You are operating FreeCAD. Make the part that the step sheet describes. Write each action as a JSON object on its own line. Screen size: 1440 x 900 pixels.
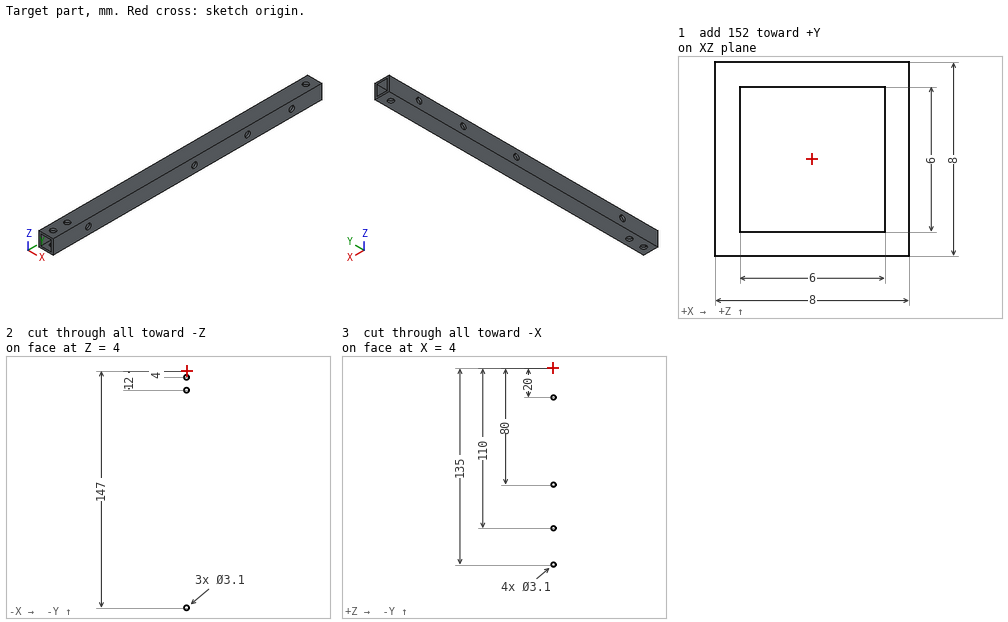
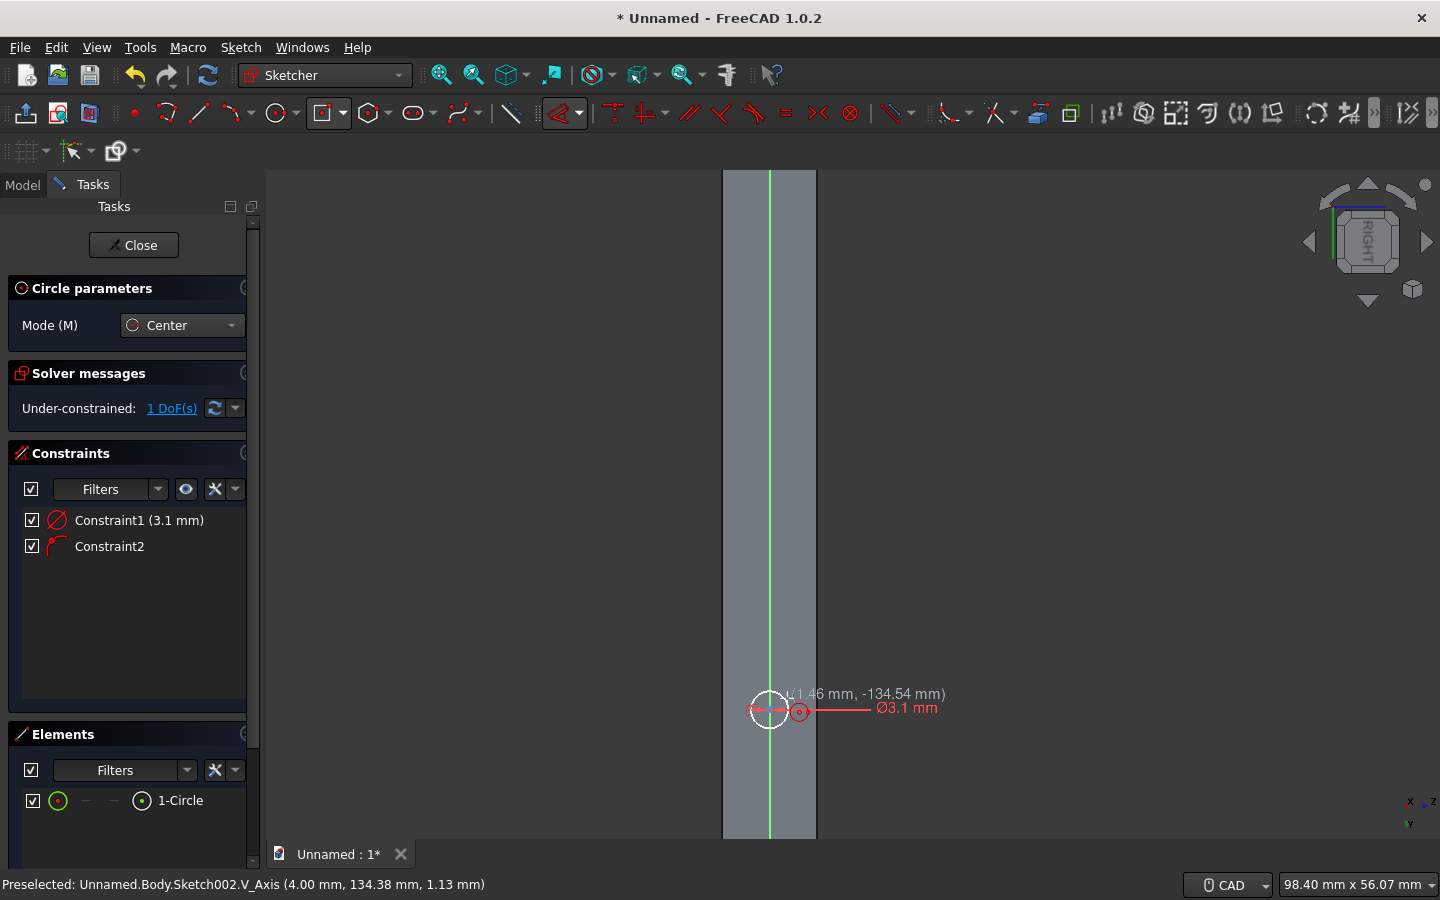
{"action": "scroll", "coordinate": [789, 700], "scroll_direction": "down", "scroll_amount": 7}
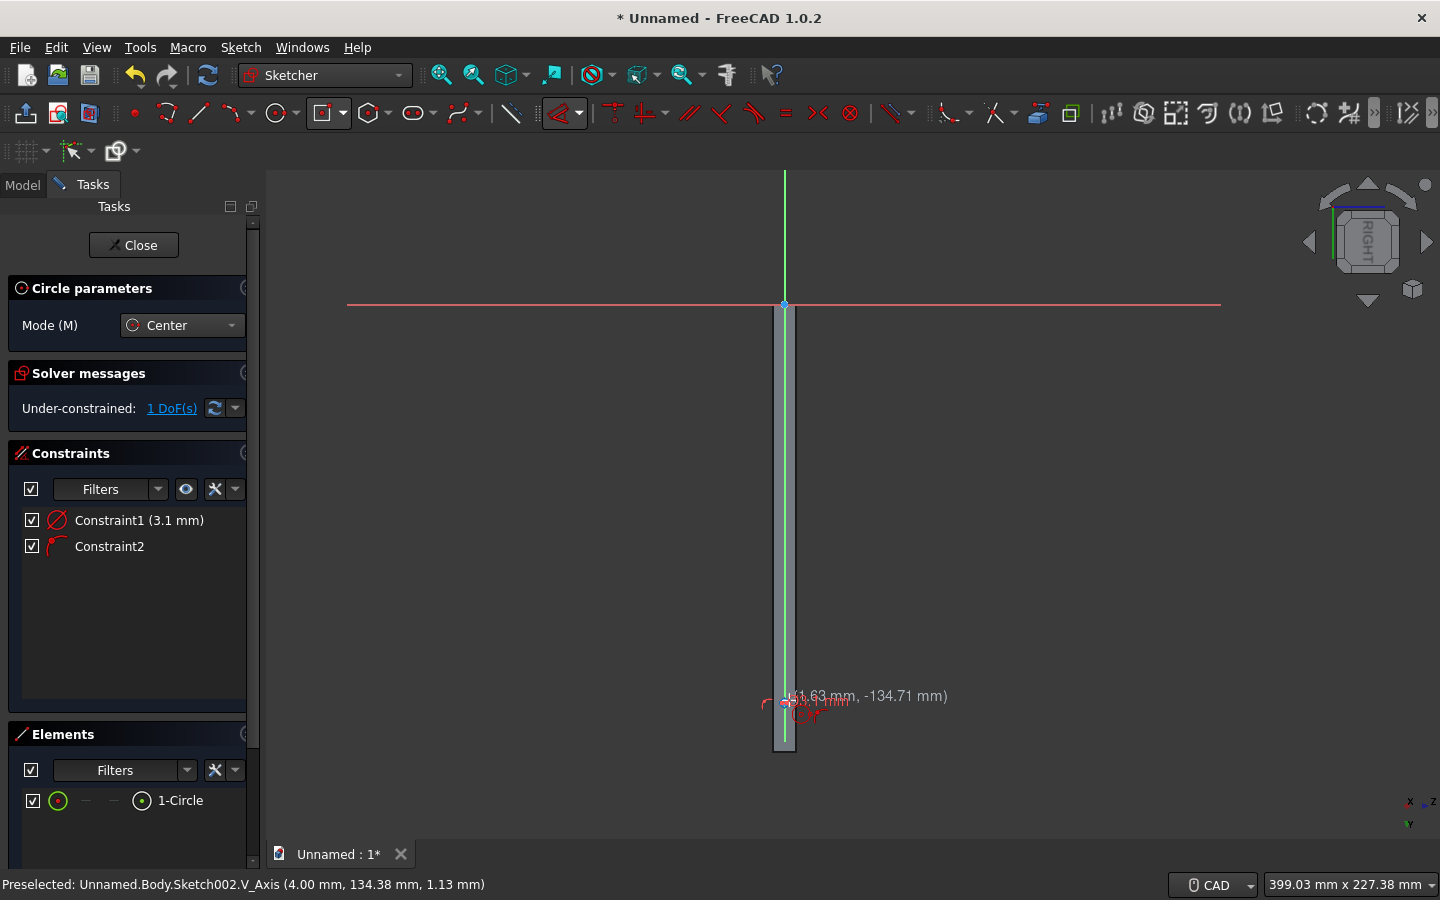
{"action": "scroll", "coordinate": [785, 363], "scroll_direction": "up", "scroll_amount": 9}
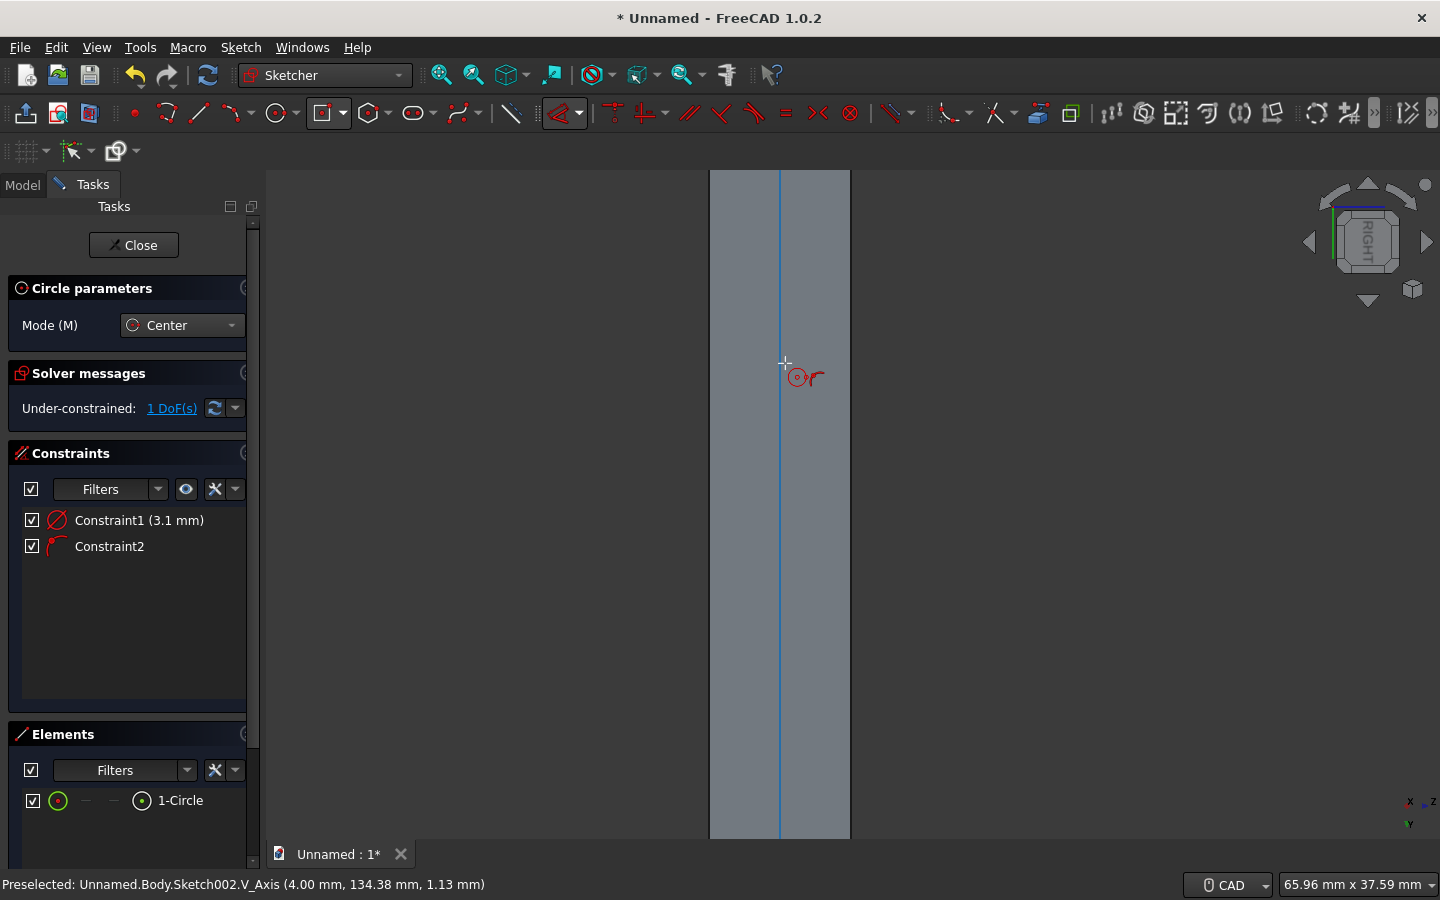
{"action": "scroll", "coordinate": [785, 362], "scroll_direction": "down", "scroll_amount": 9}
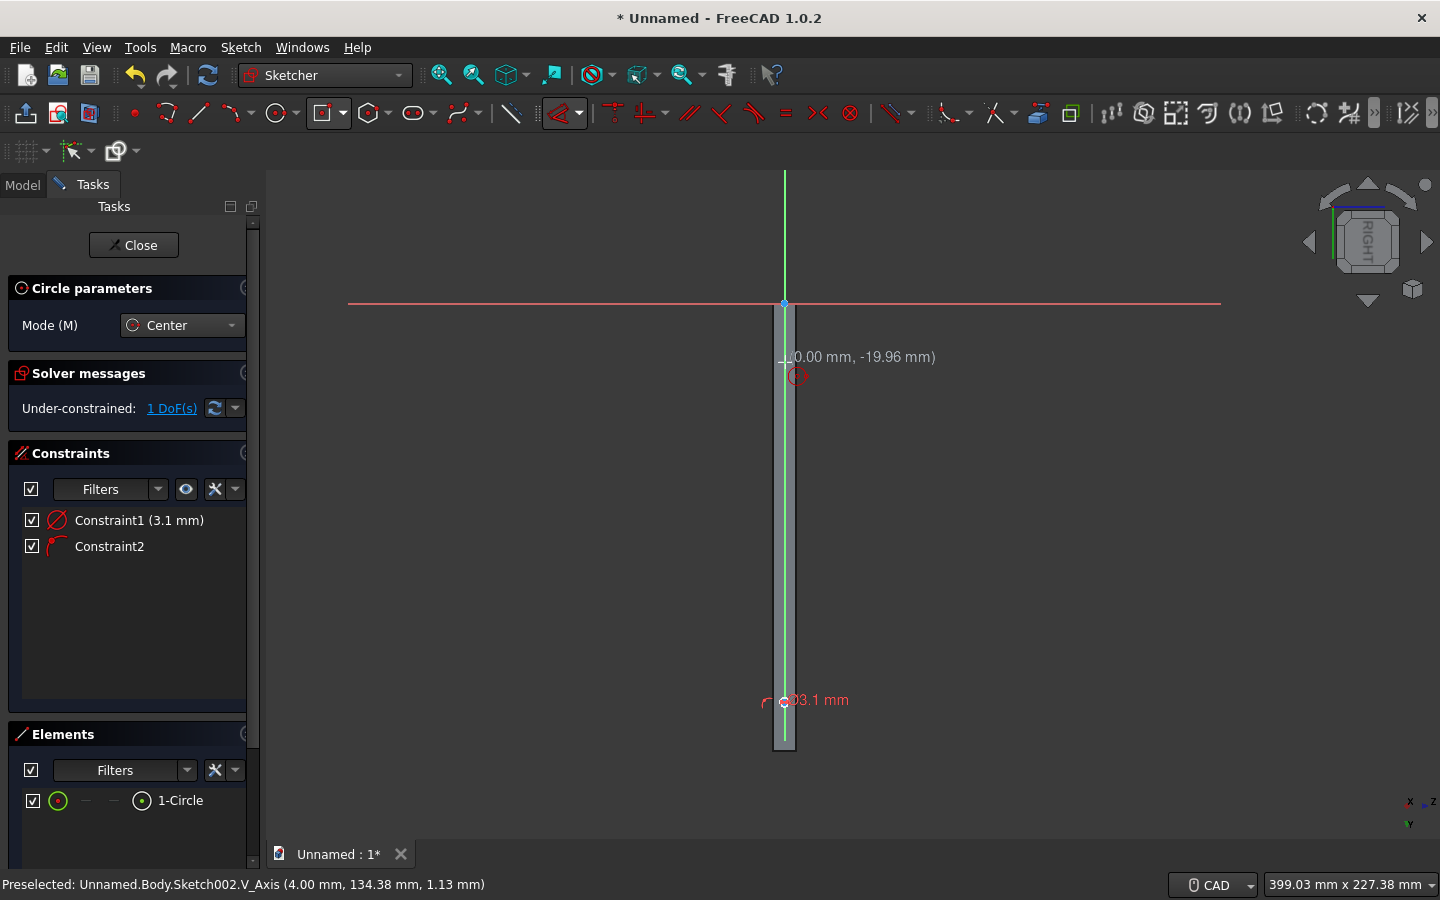
{"action": "left_click", "coordinate": [785, 363]}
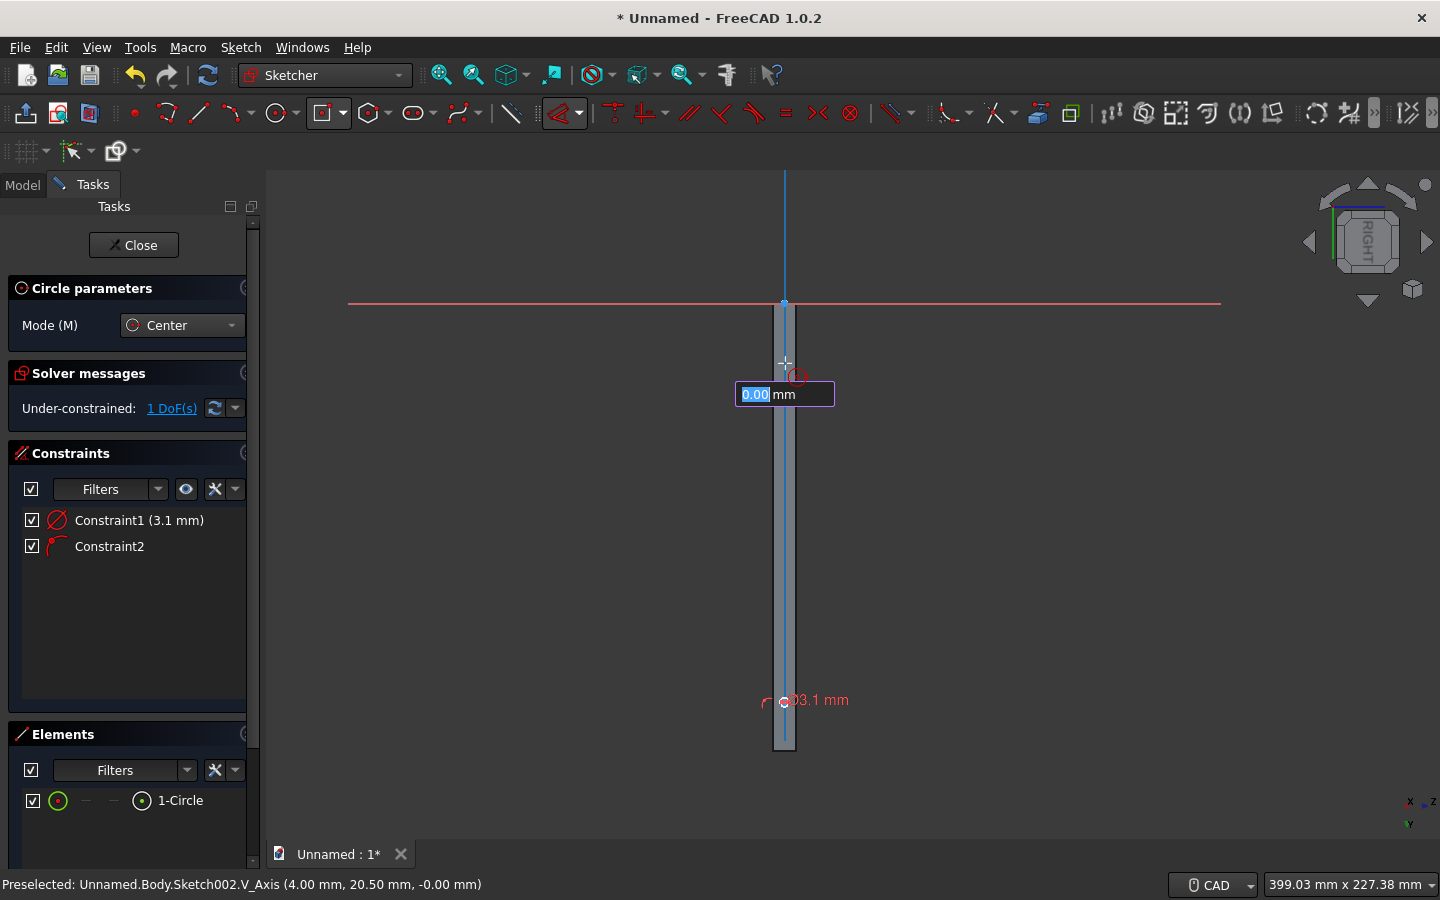
{"action": "scroll", "coordinate": [789, 361], "scroll_direction": "up", "scroll_amount": 7}
{"action": "mouse_move", "coordinate": [787, 360]}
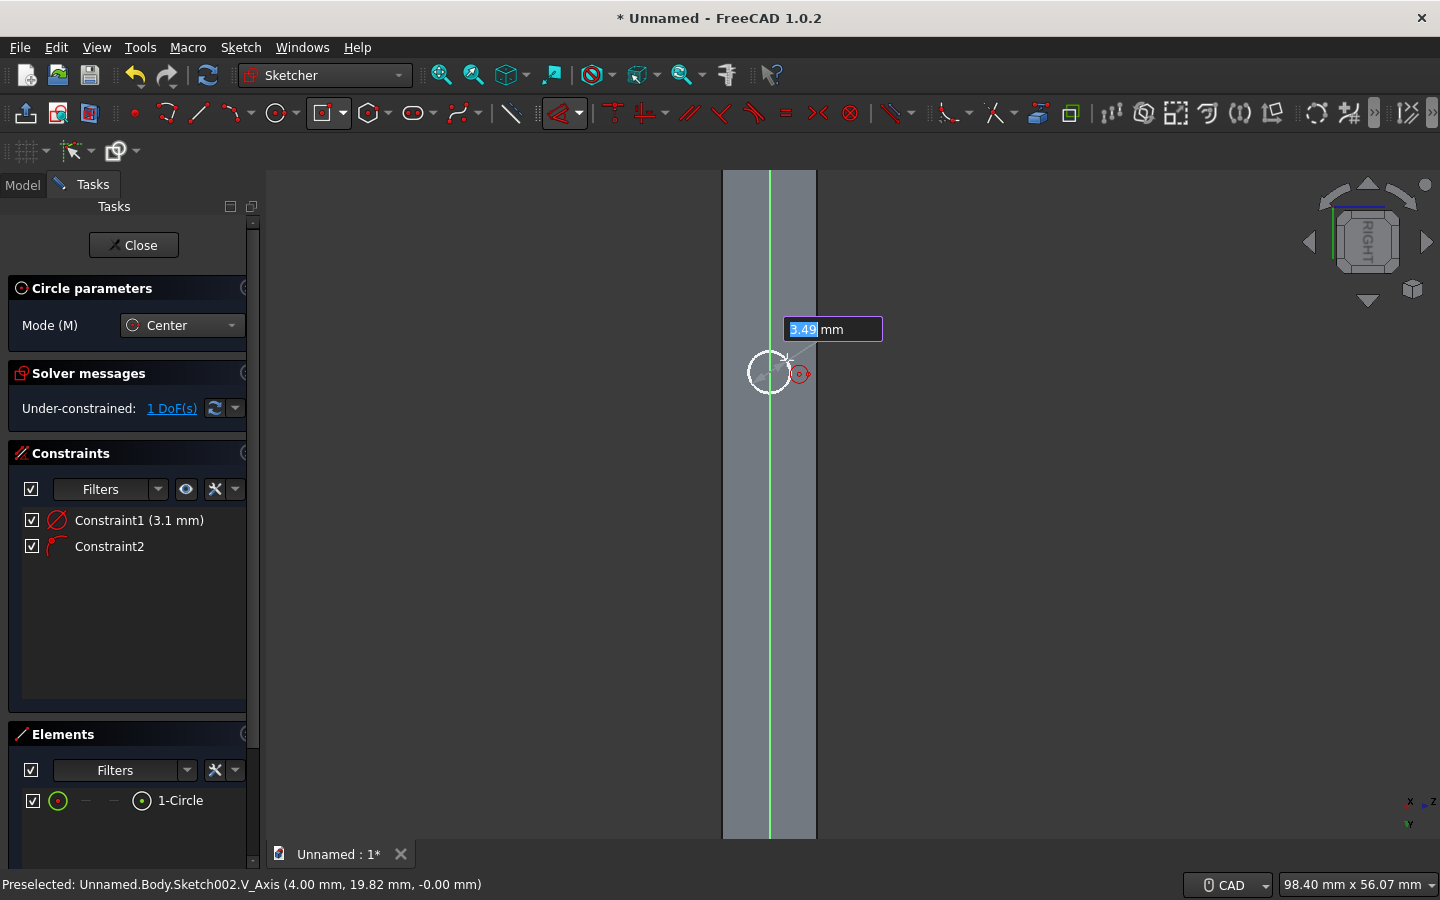
{"action": "type", "text": "3.1"}
{"action": "key", "text": "Return"}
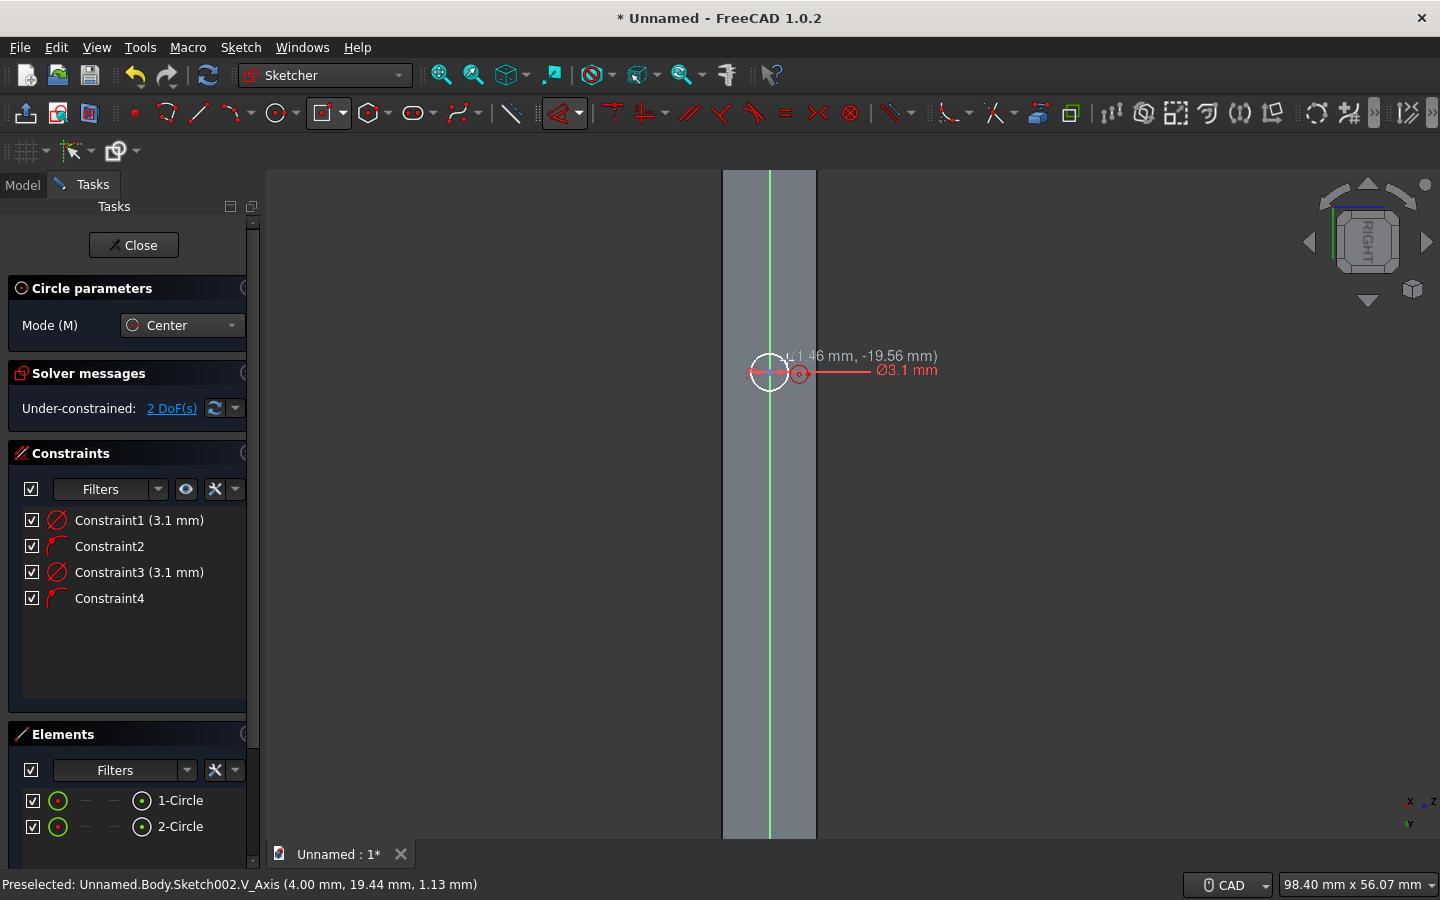
{"action": "scroll", "coordinate": [789, 361], "scroll_direction": "down", "scroll_amount": 7}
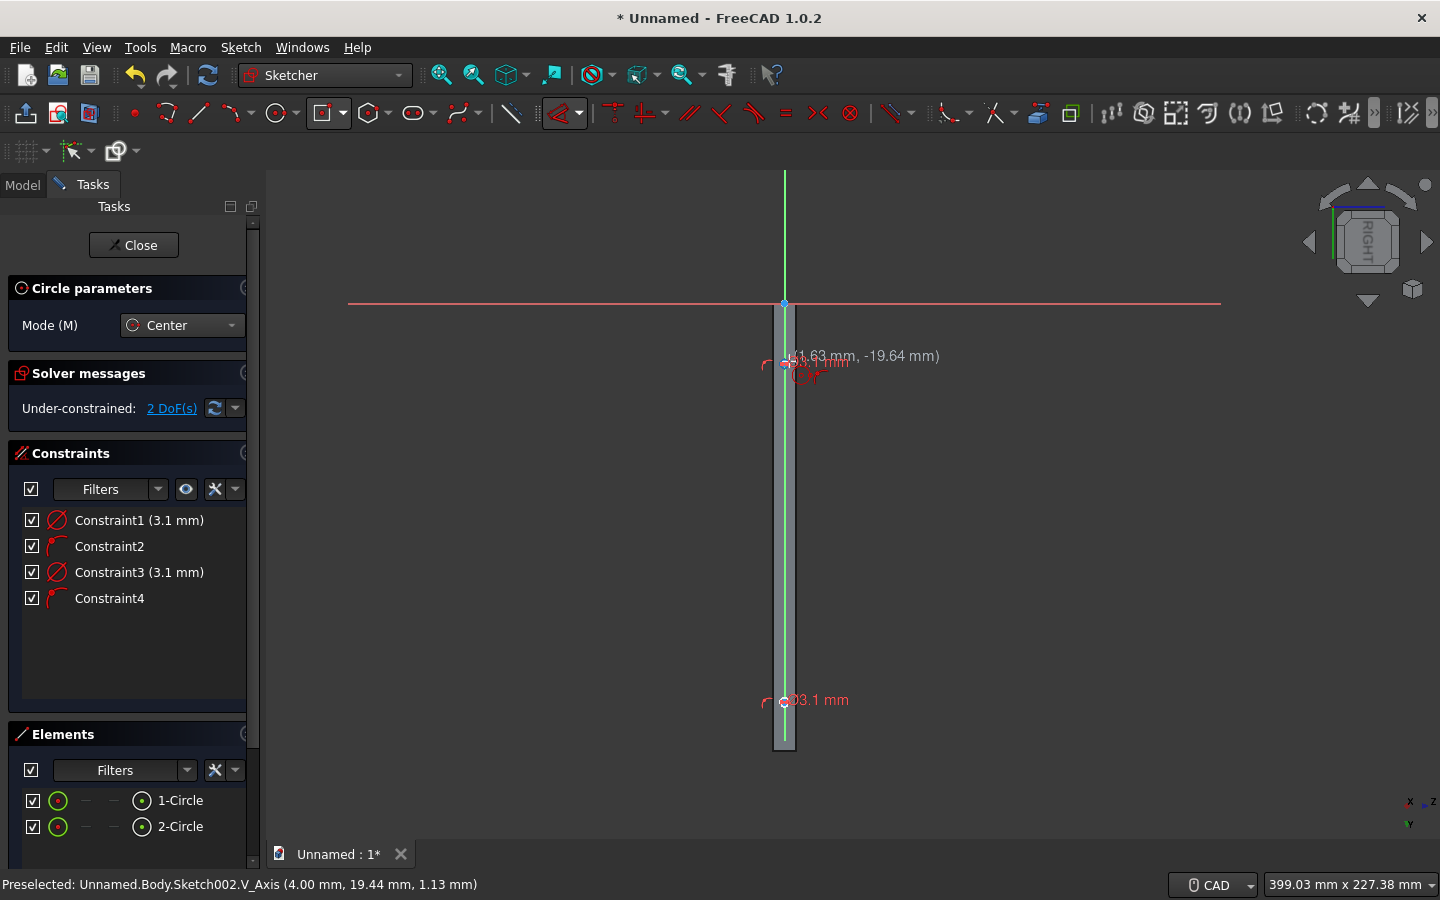
{"action": "scroll", "coordinate": [785, 627], "scroll_direction": "up", "scroll_amount": 9}